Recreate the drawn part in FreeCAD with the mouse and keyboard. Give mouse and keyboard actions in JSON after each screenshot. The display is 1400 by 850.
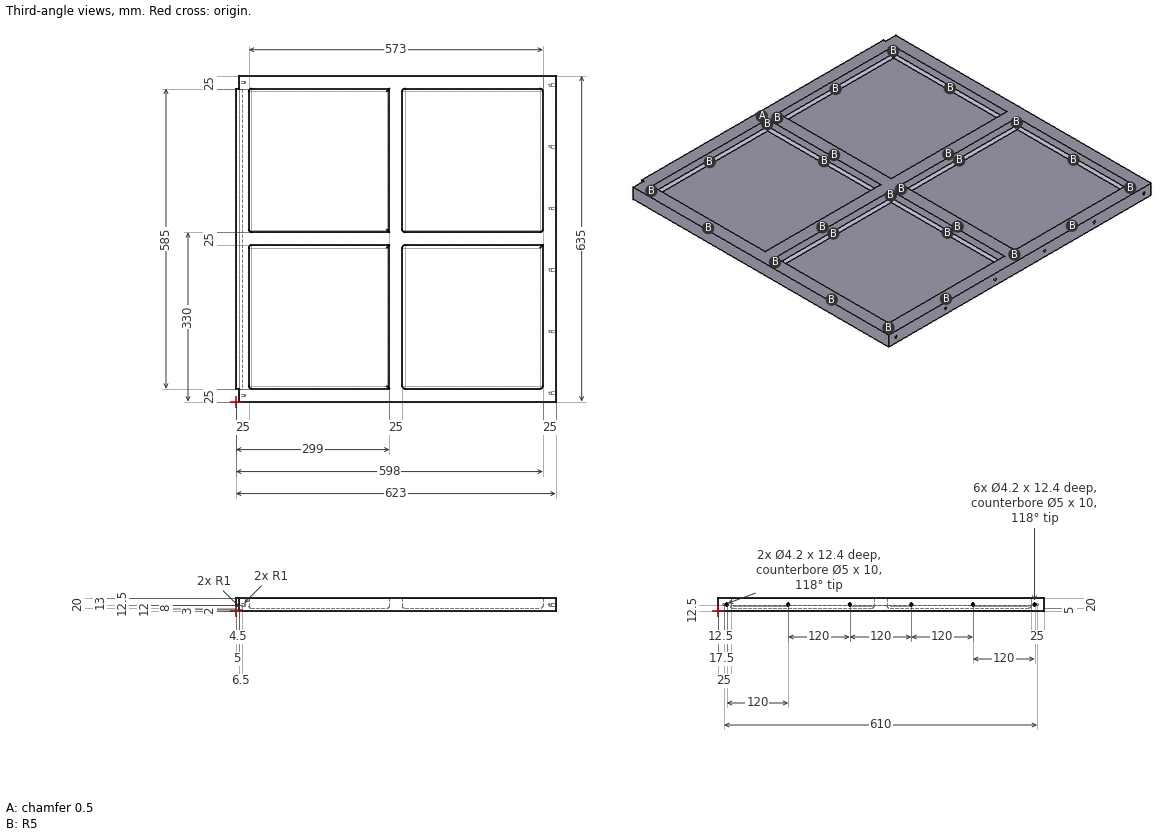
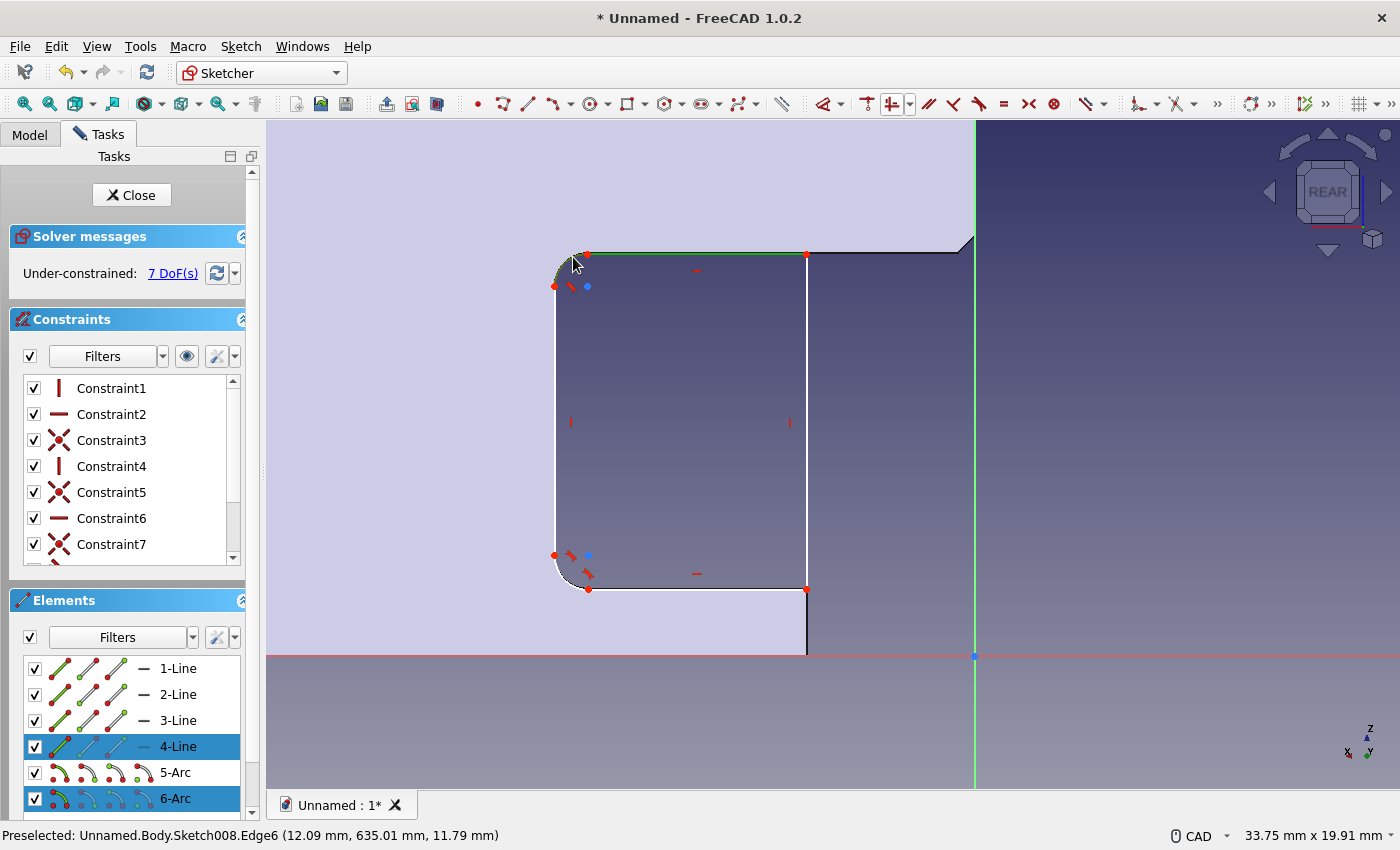
{"action": "left_click", "coordinate": [979, 104]}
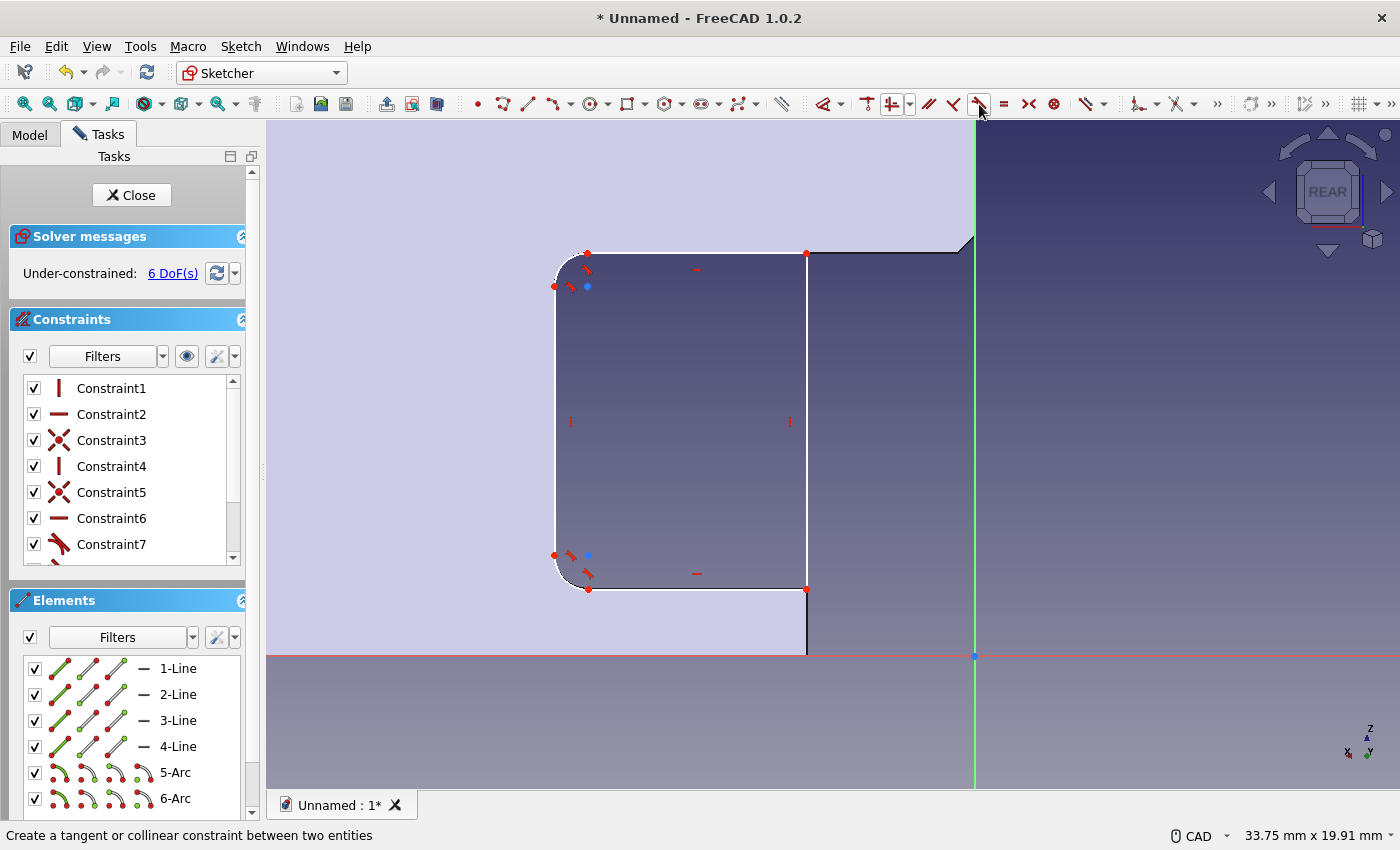
{"action": "left_click", "coordinate": [559, 571]}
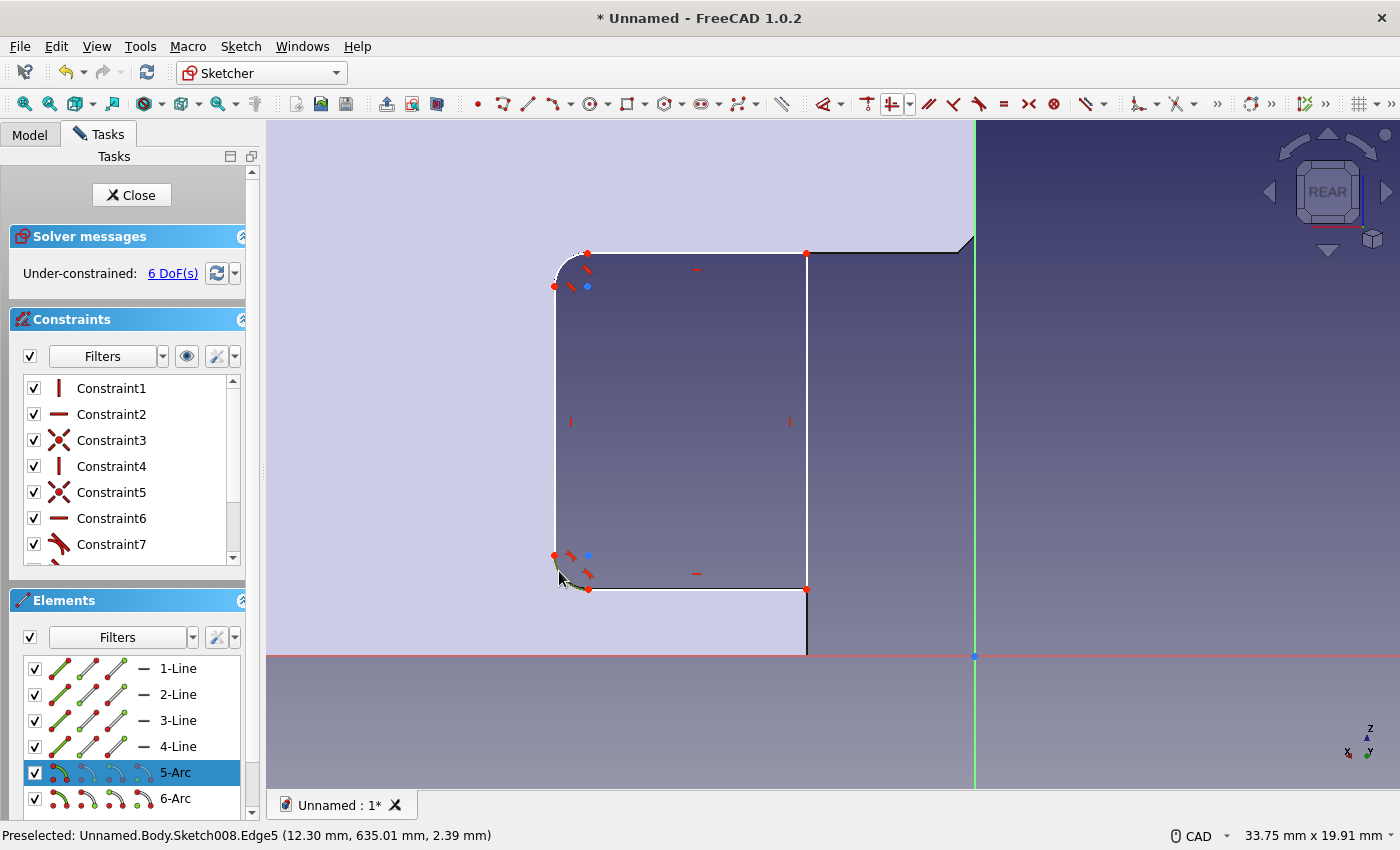
{"action": "left_click", "coordinate": [573, 257]}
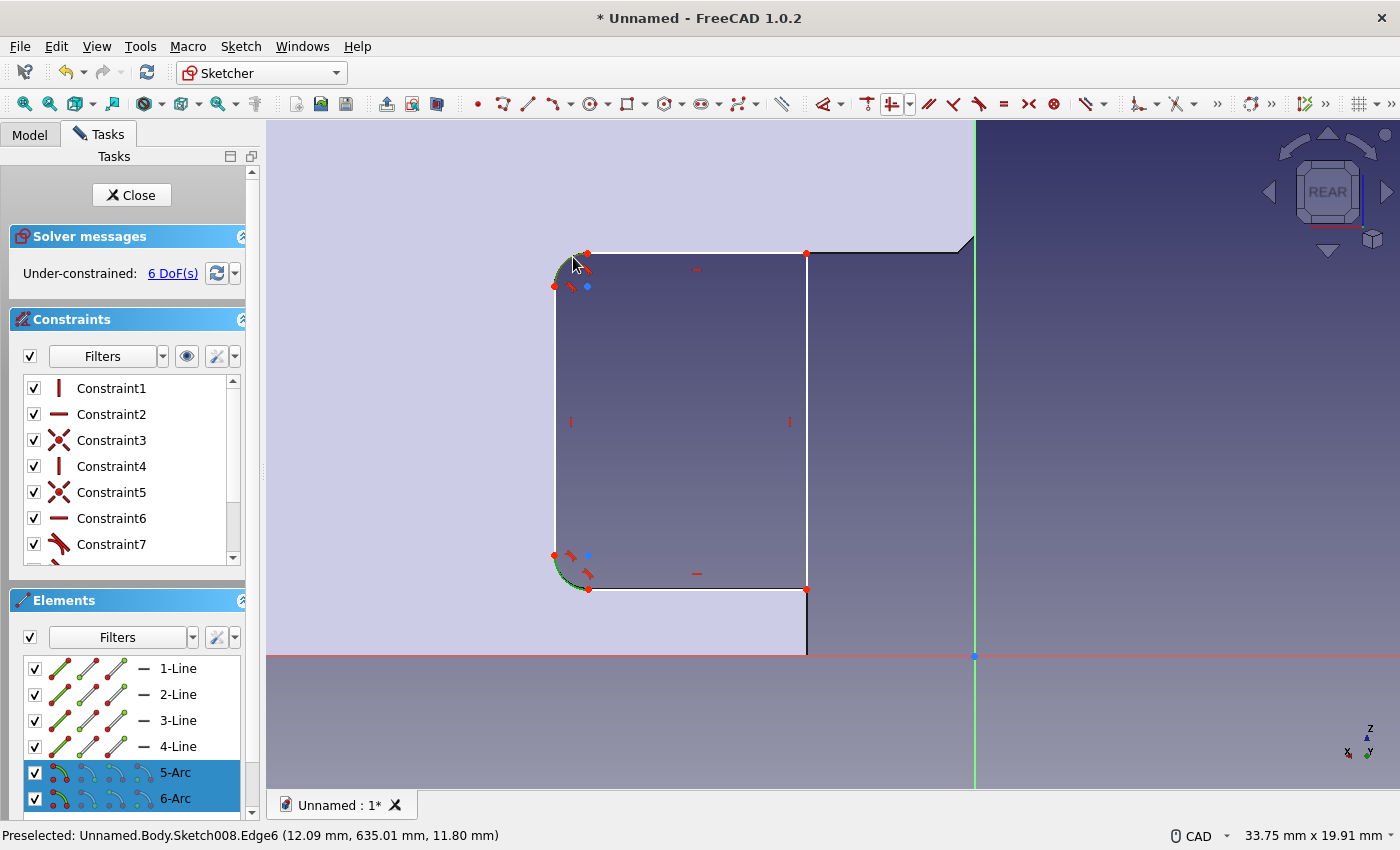
{"action": "left_click", "coordinate": [1004, 104]}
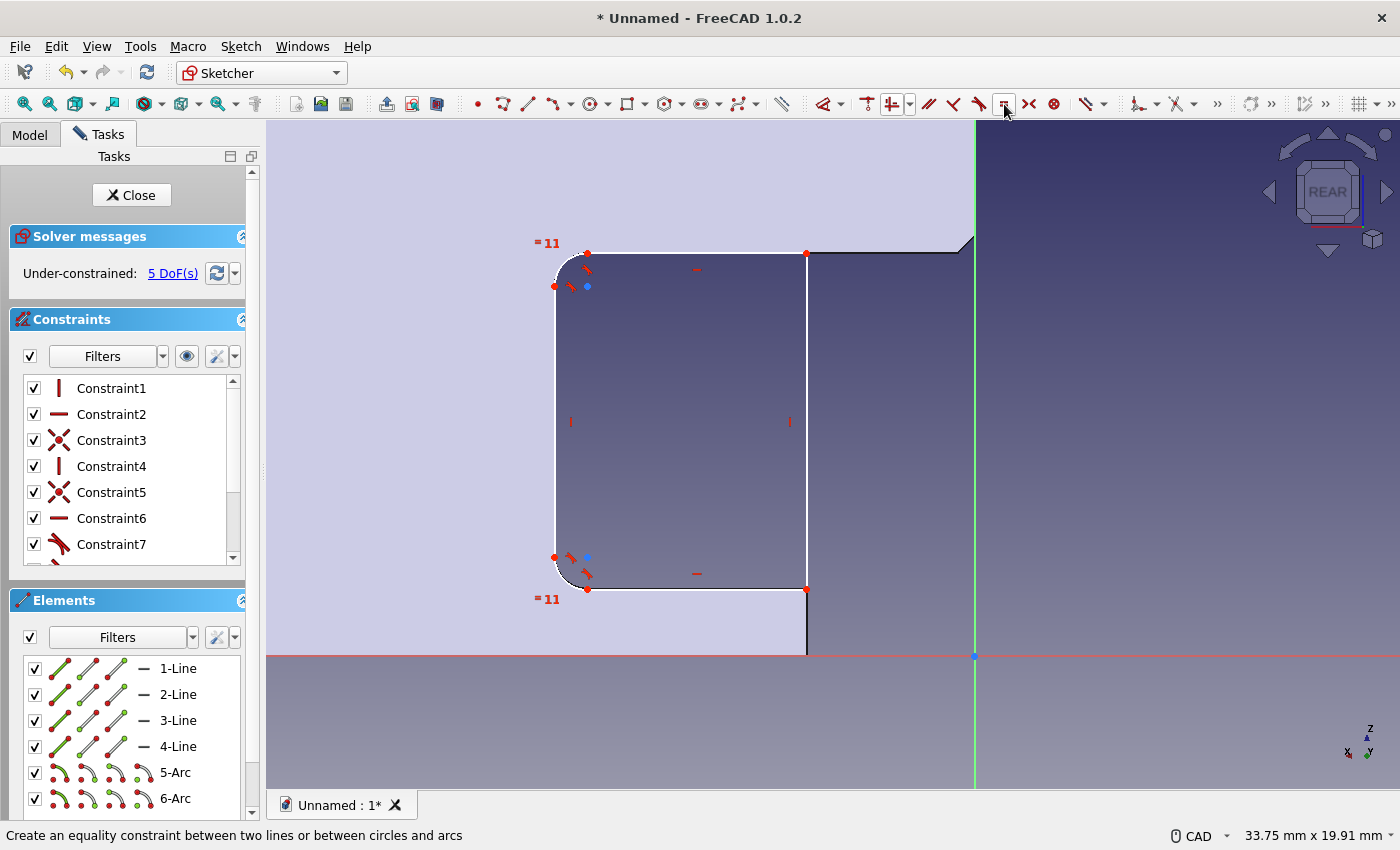
{"action": "left_click", "coordinate": [822, 104]}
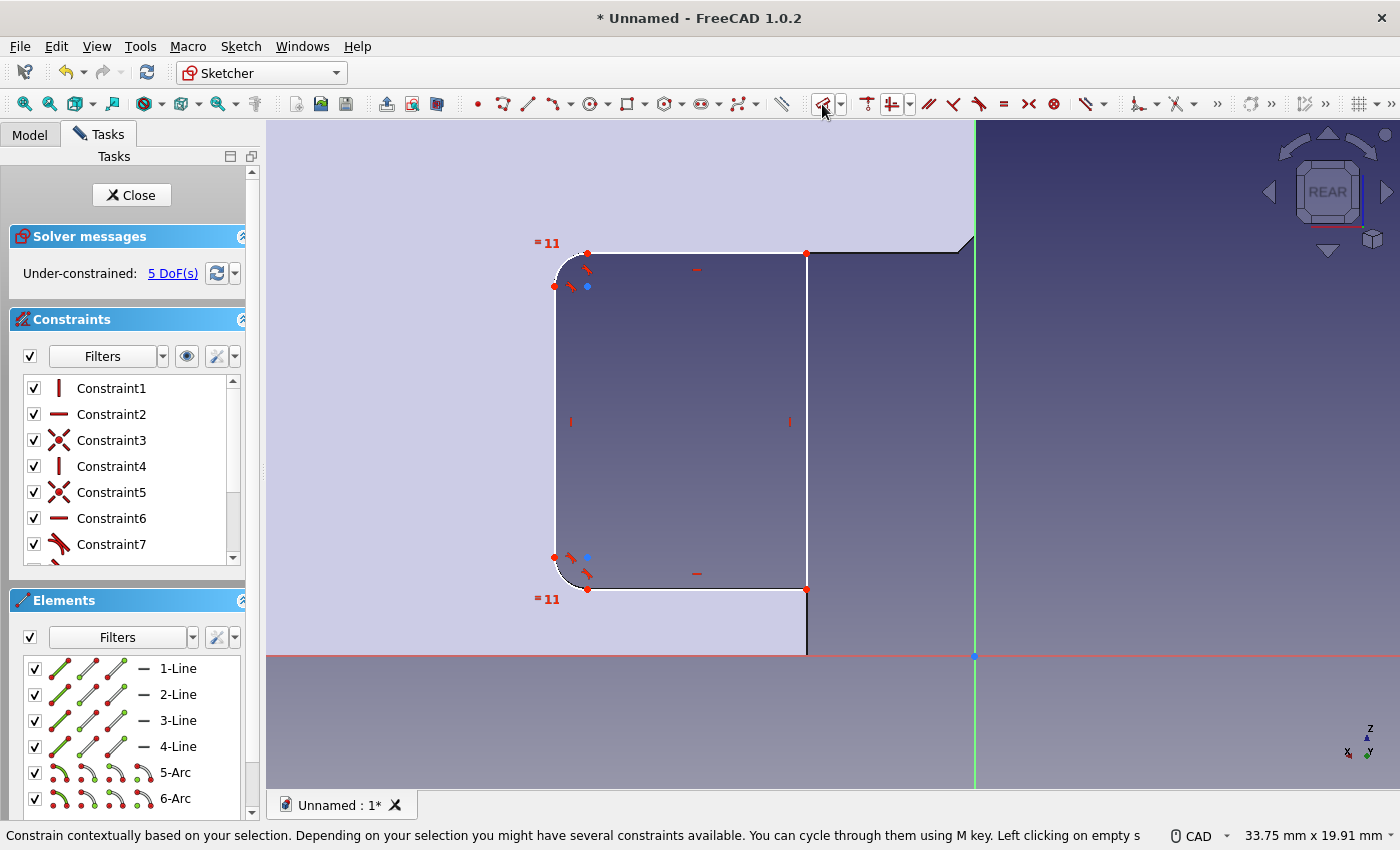
{"action": "left_click", "coordinate": [558, 572]}
{"action": "left_click", "coordinate": [529, 586]}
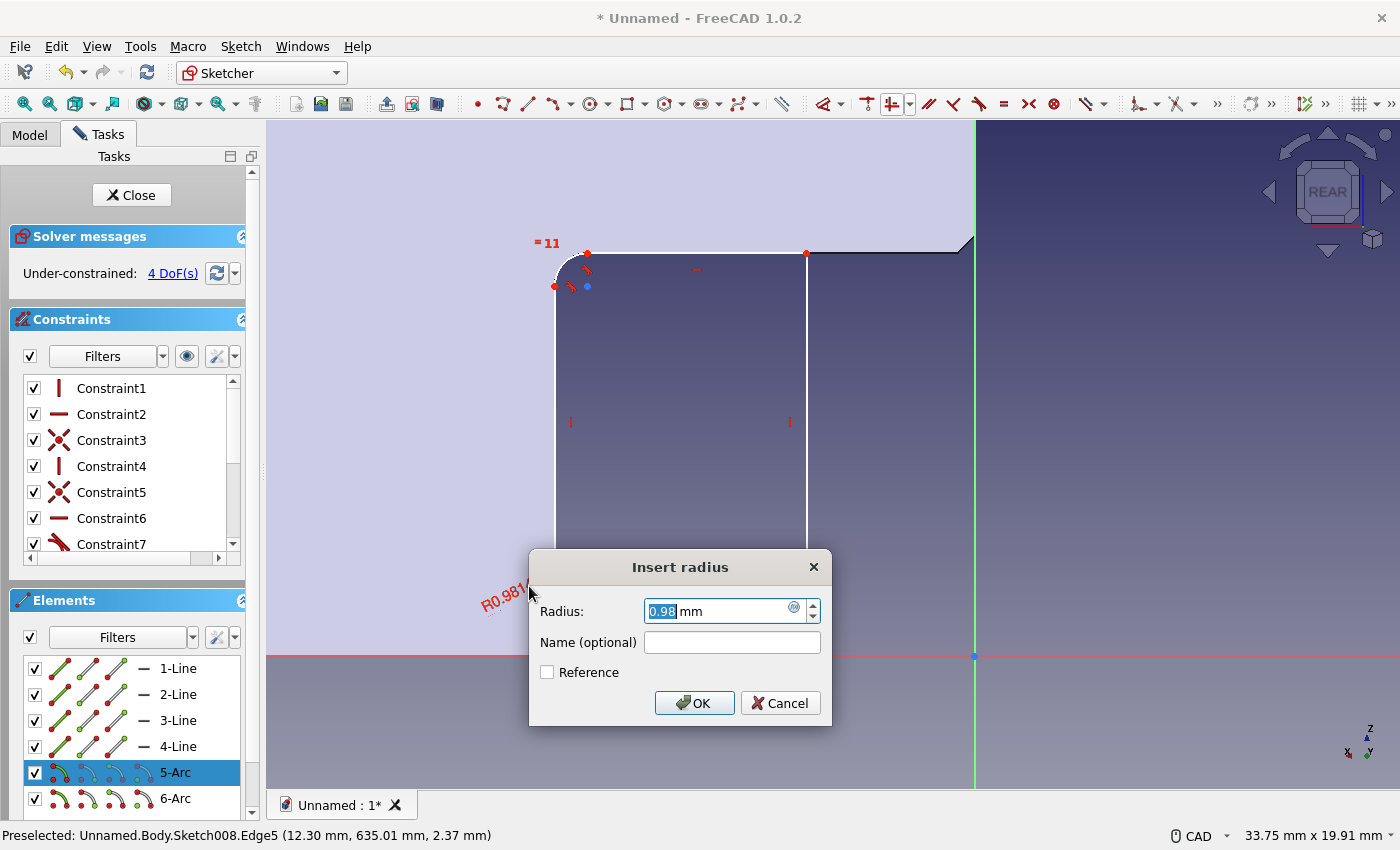
{"action": "type", "text": "1"}
{"action": "key", "text": "Return"}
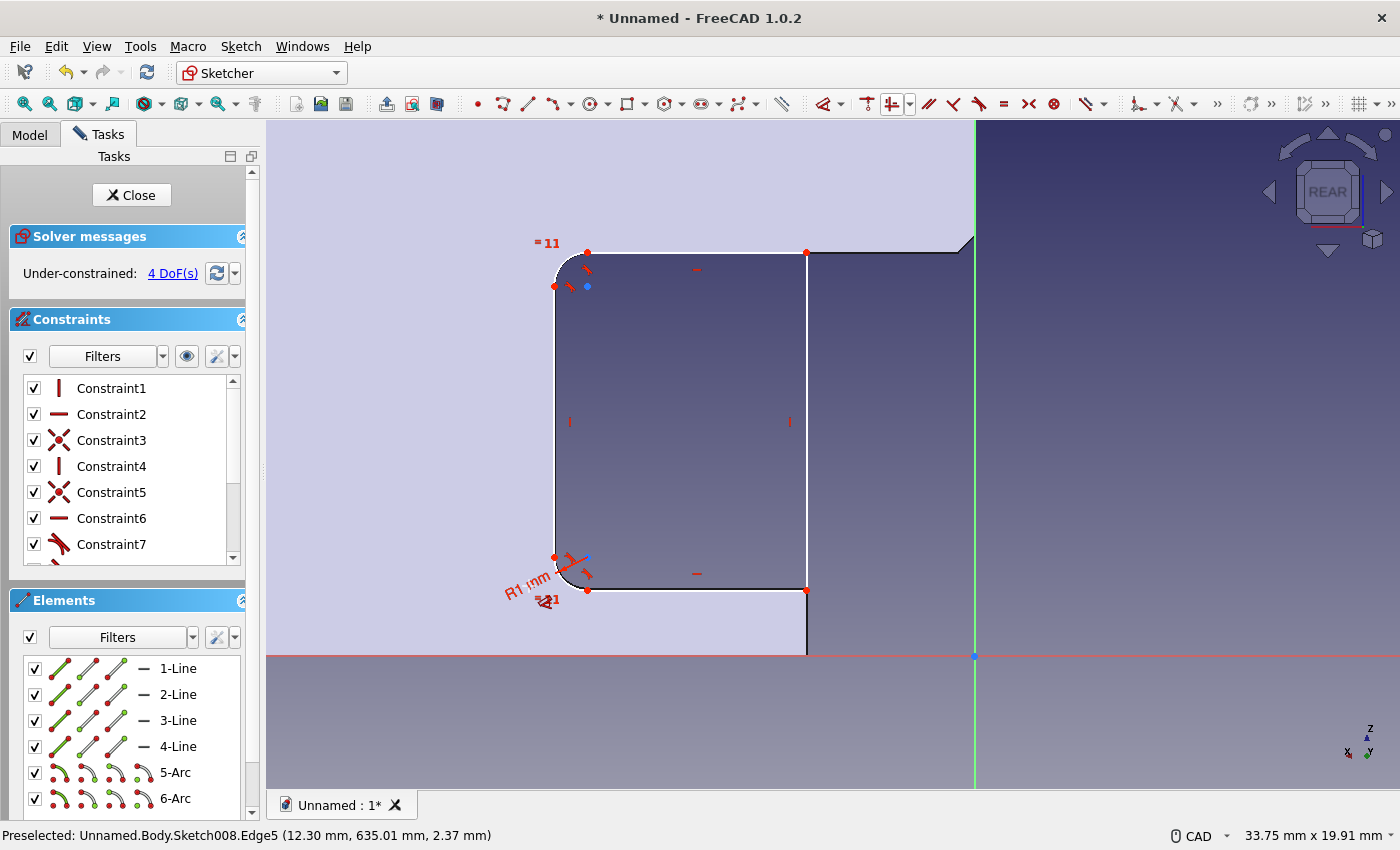
{"action": "left_click", "coordinate": [554, 367]}
{"action": "left_click", "coordinate": [520, 422]}